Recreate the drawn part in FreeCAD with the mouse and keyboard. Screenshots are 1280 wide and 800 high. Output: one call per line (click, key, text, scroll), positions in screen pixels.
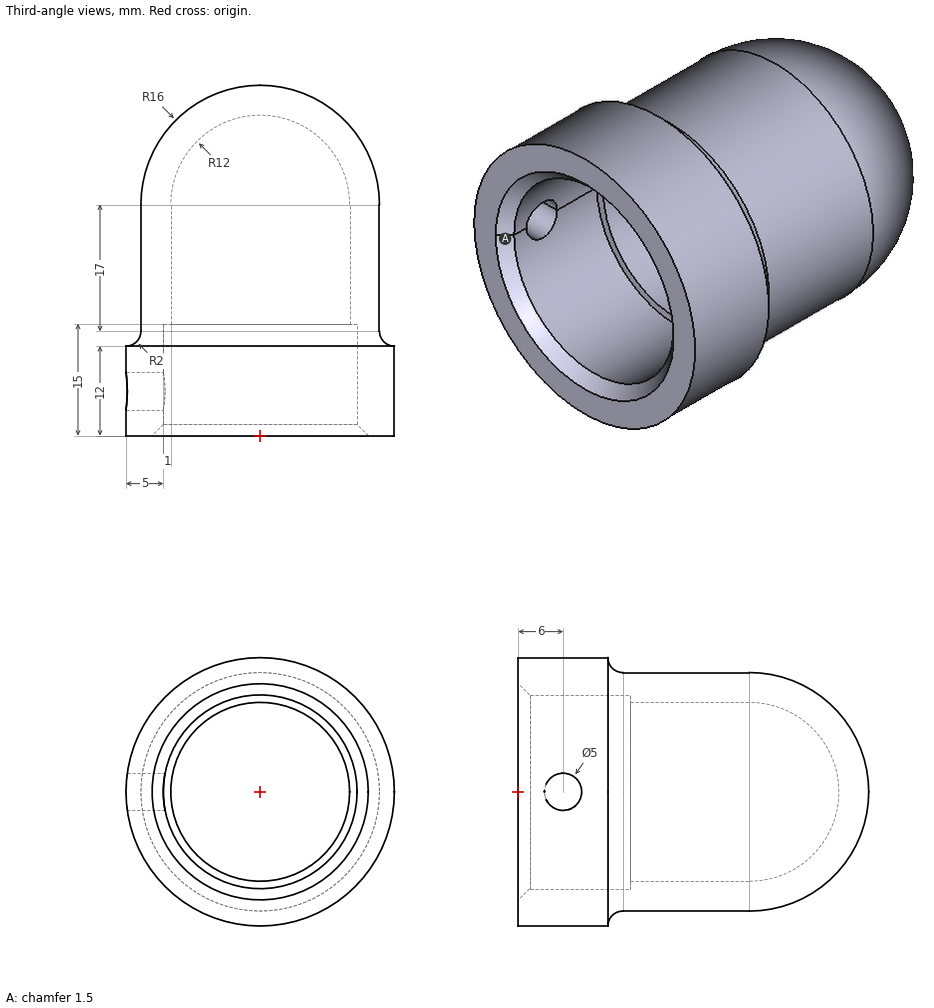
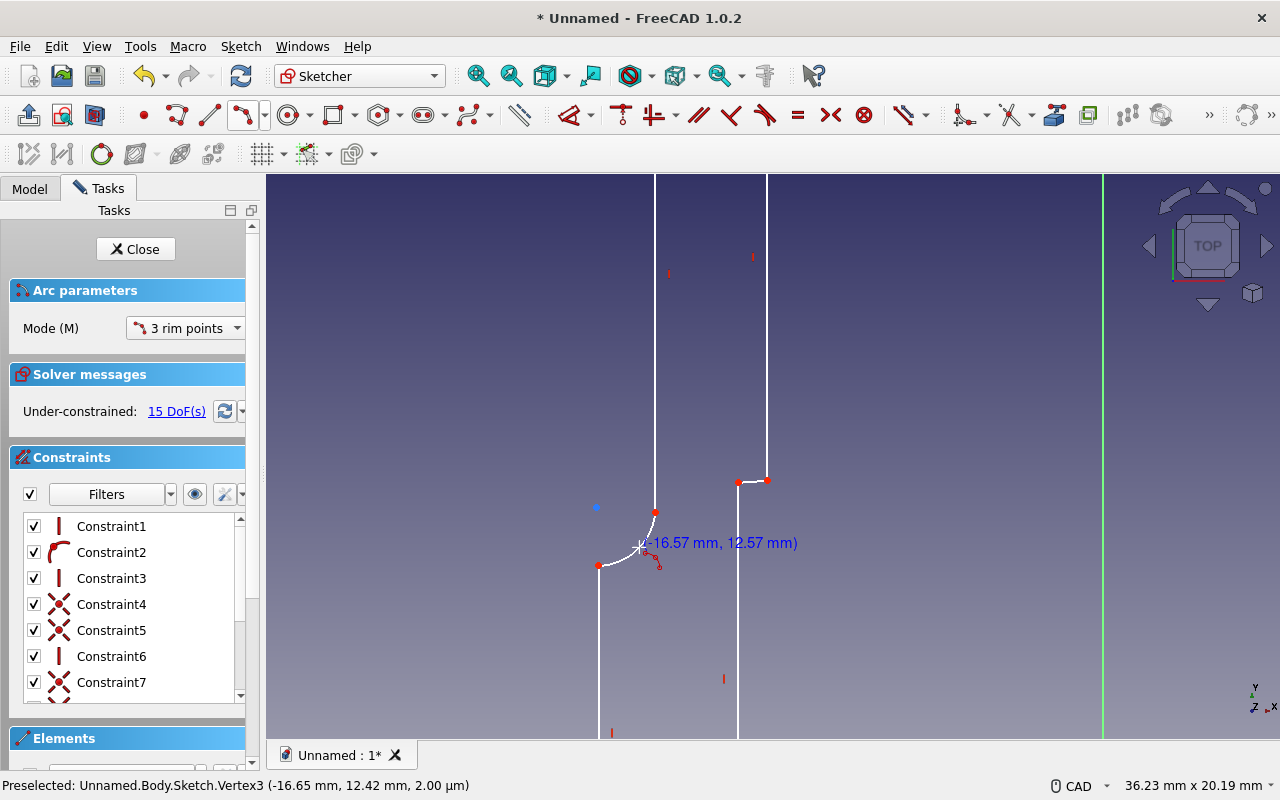
scroll(641, 549, down, 6)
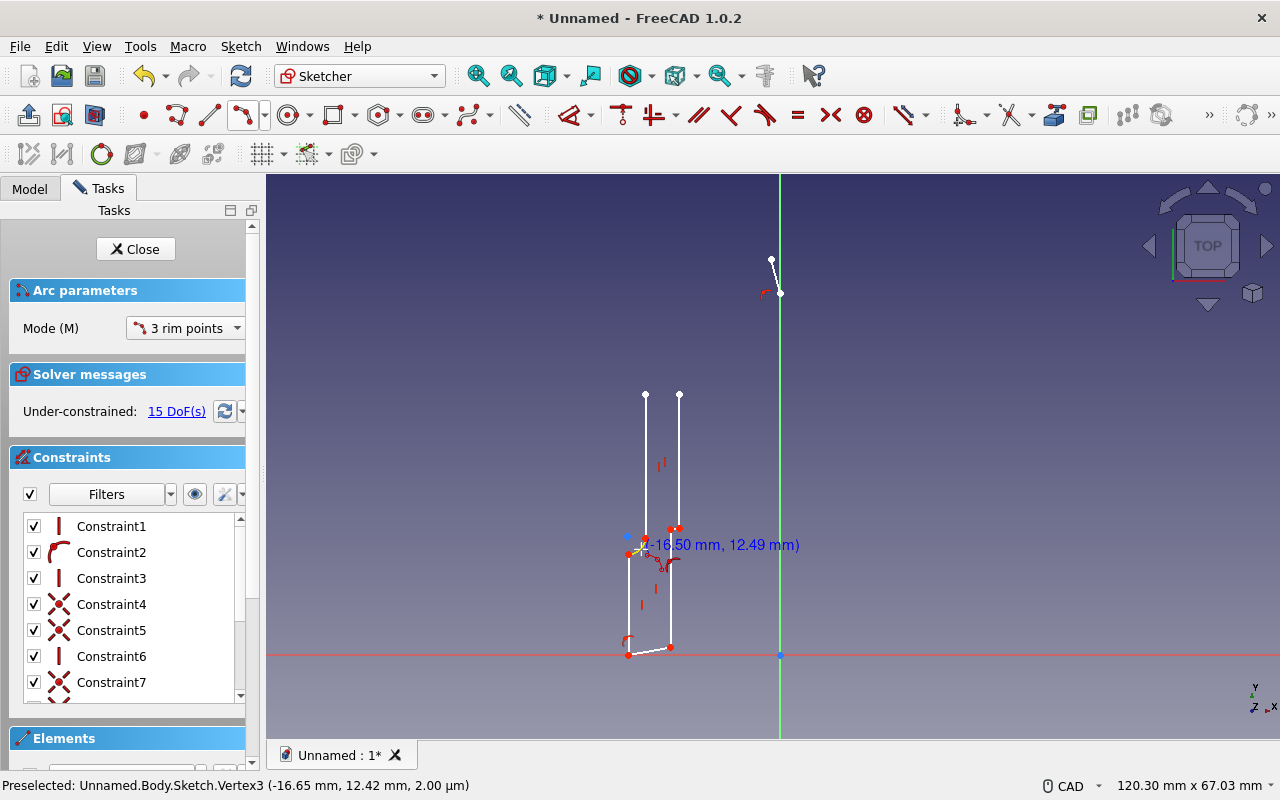
click(679, 394)
click(780, 294)
click(709, 322)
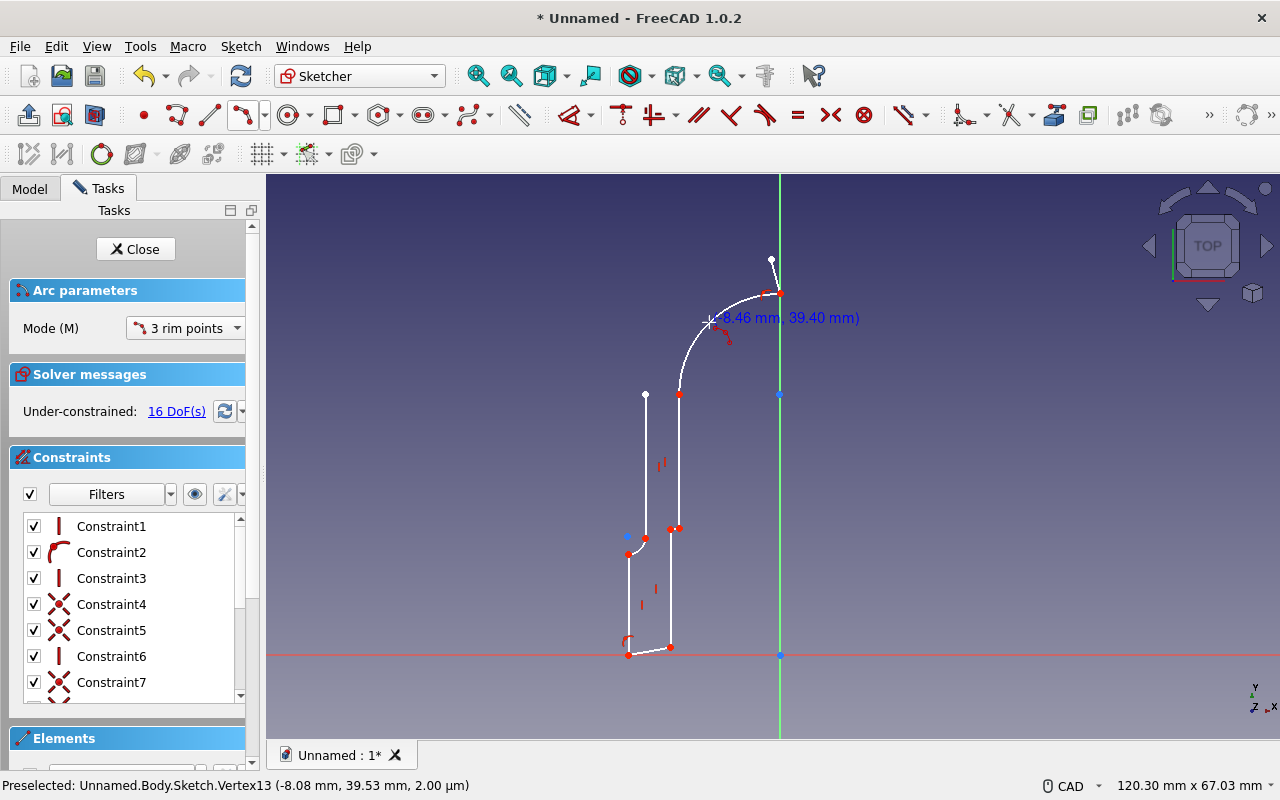
click(771, 260)
click(646, 395)
click(685, 298)
key(Escape)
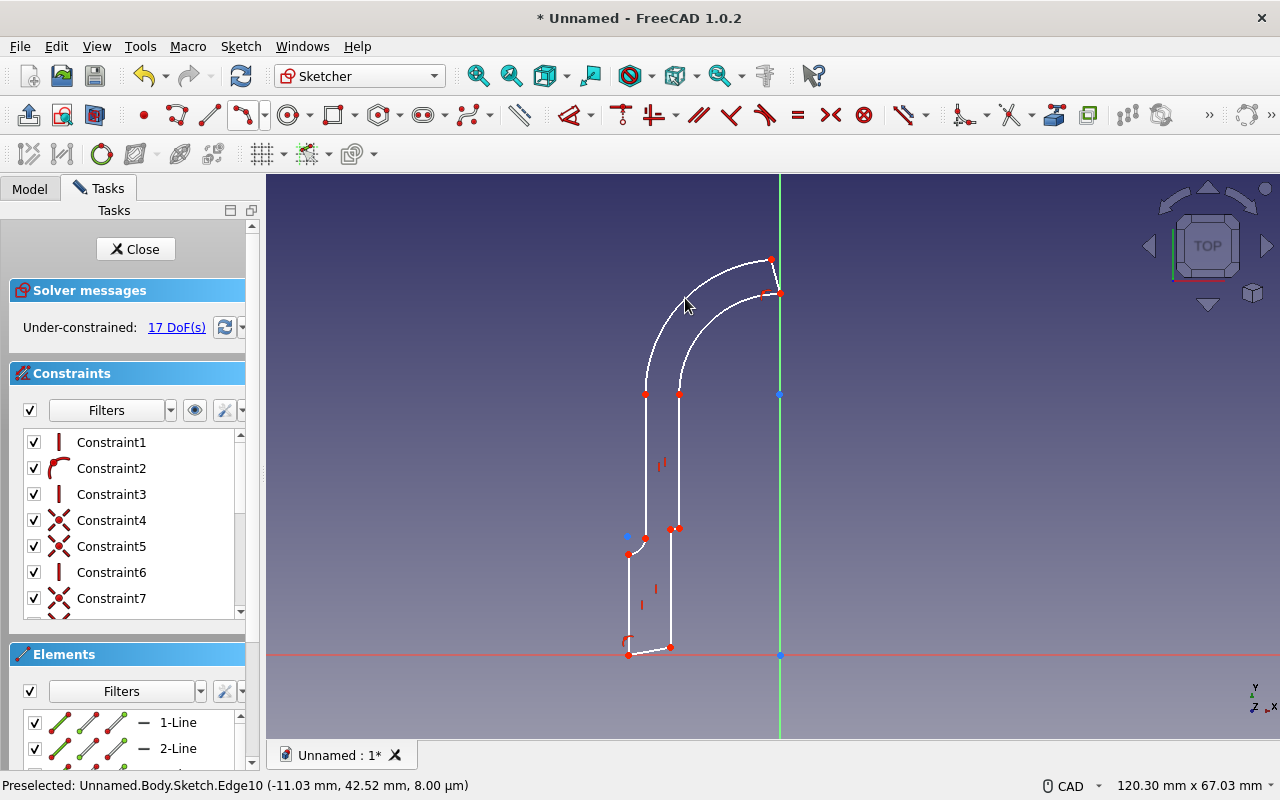
click(646, 438)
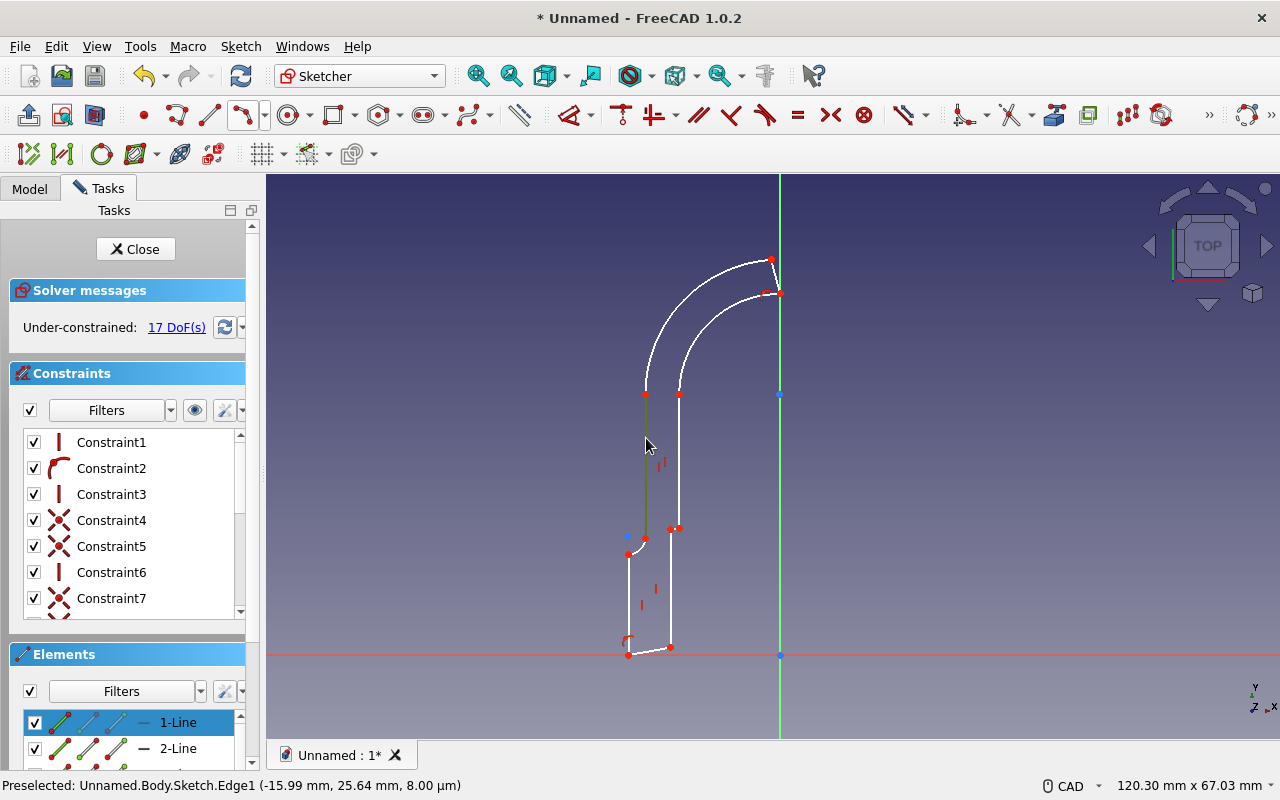
click(640, 550)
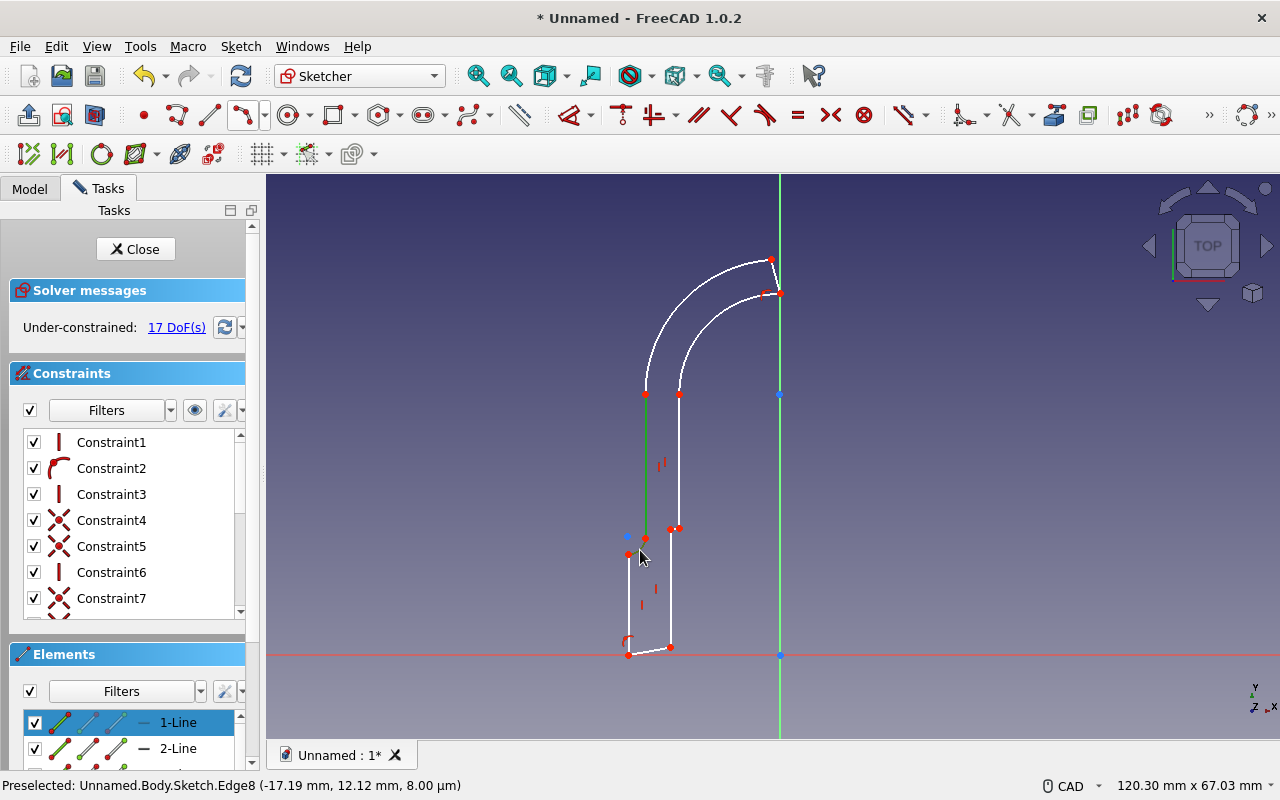
click(765, 116)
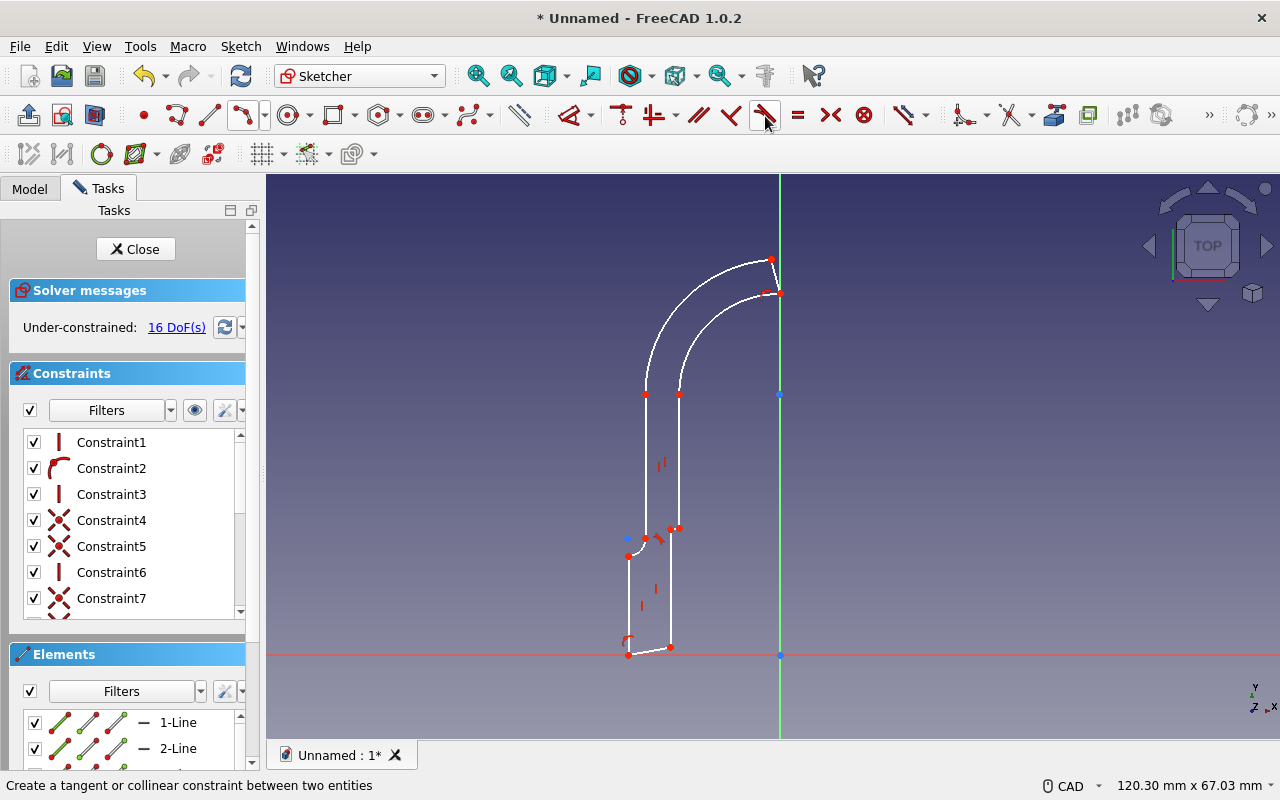
click(646, 438)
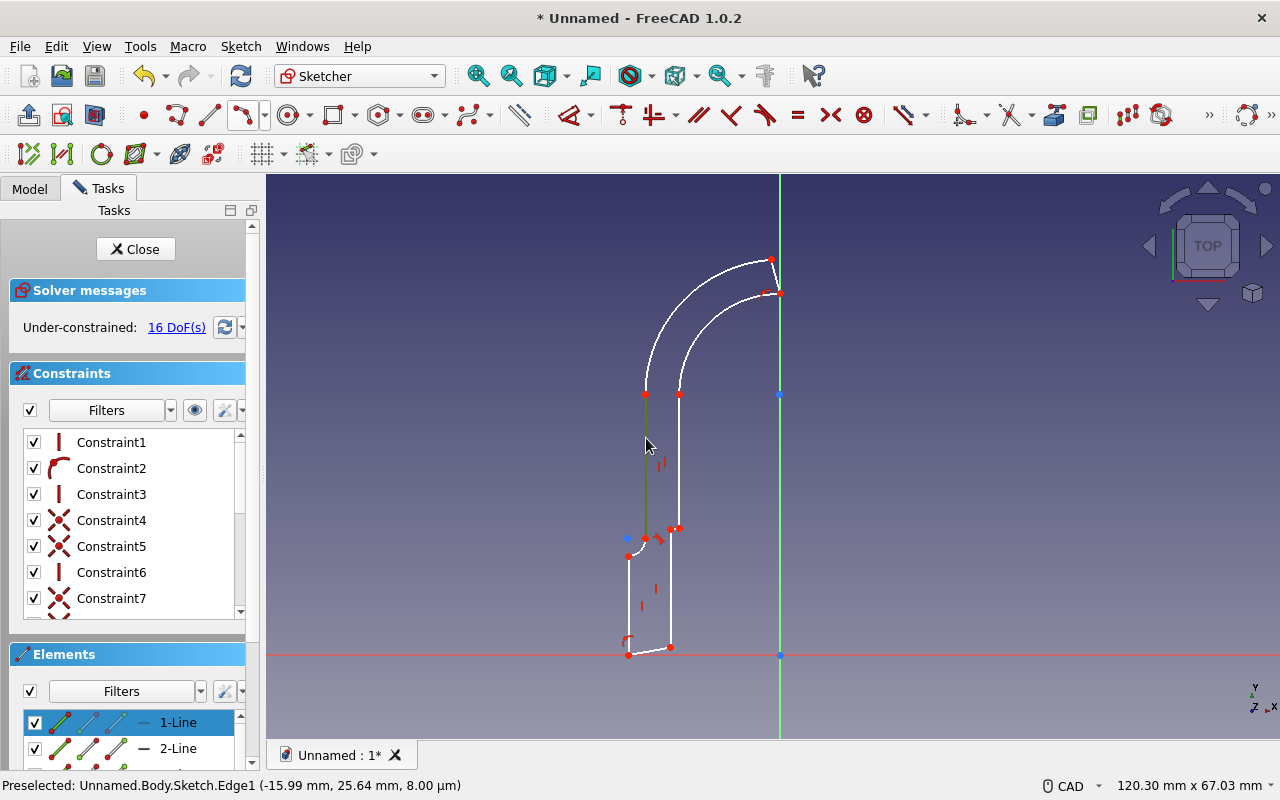
click(713, 277)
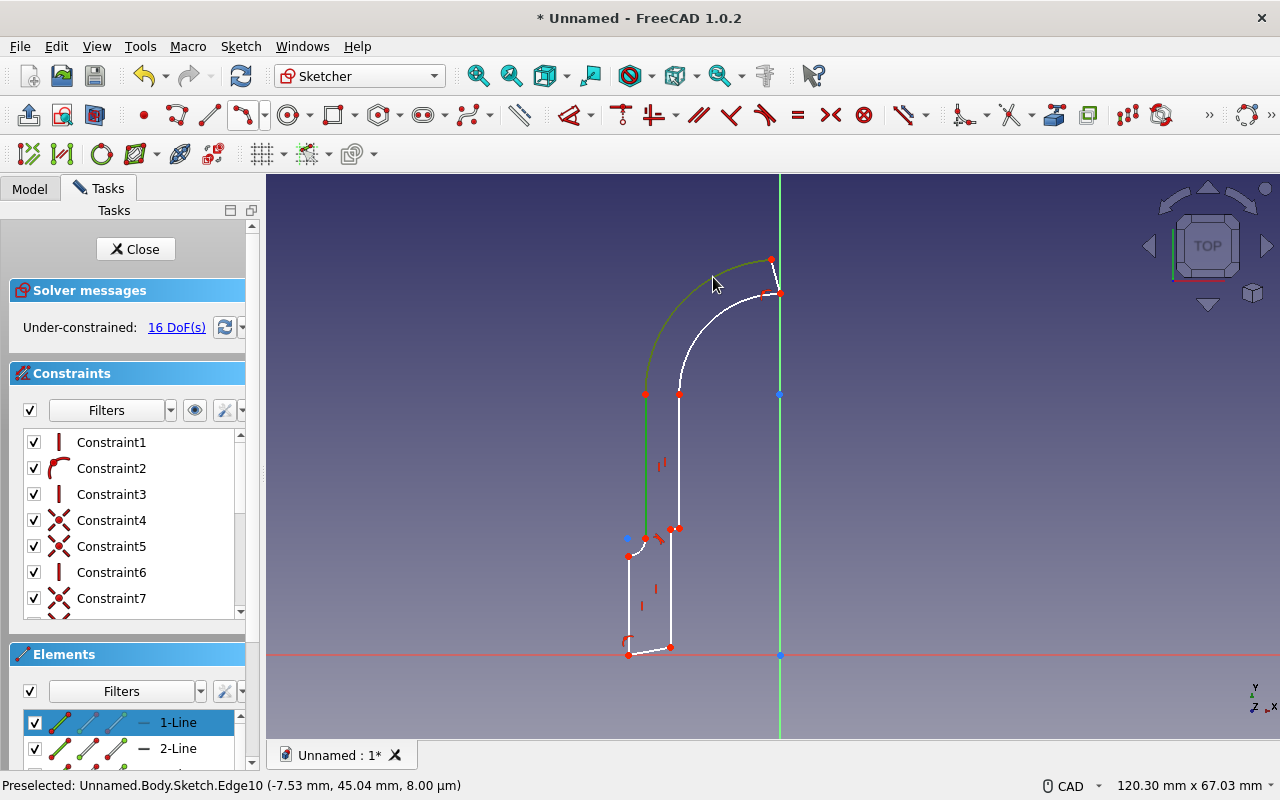
key(t)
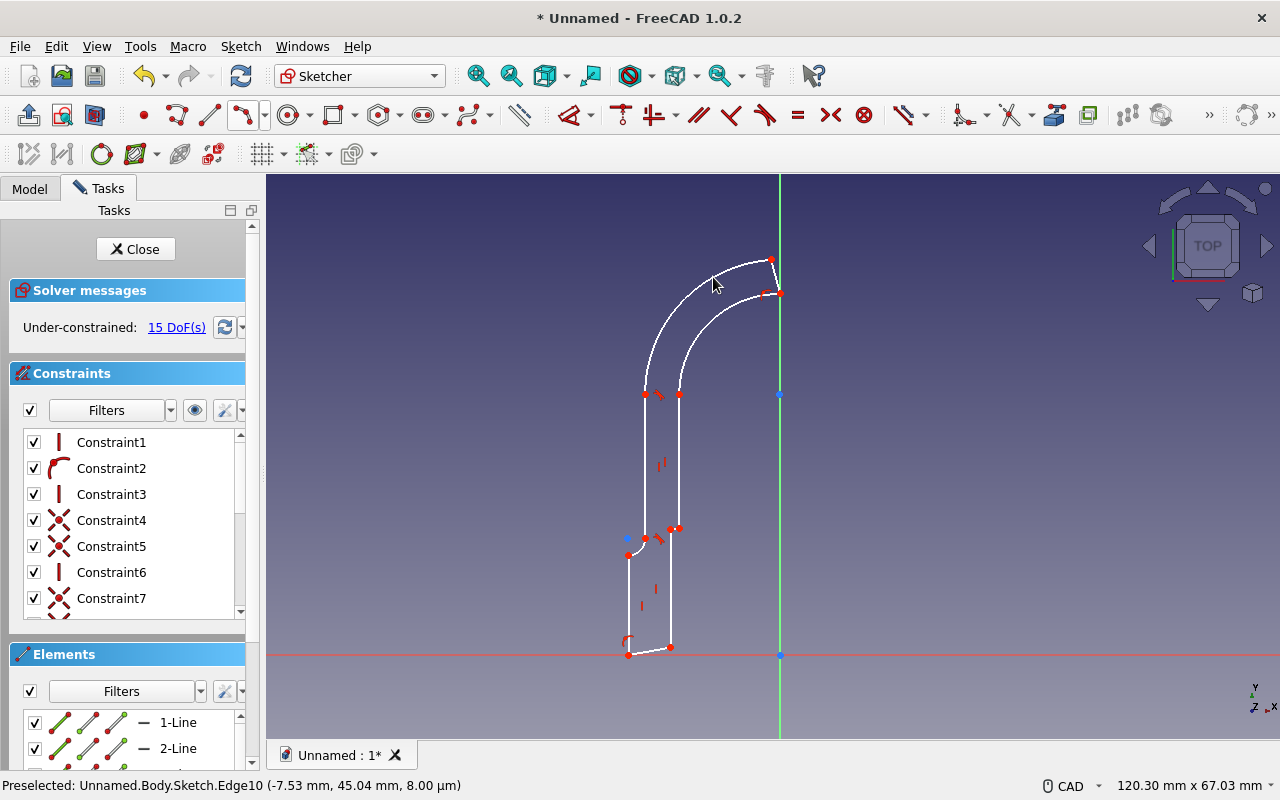
click(679, 488)